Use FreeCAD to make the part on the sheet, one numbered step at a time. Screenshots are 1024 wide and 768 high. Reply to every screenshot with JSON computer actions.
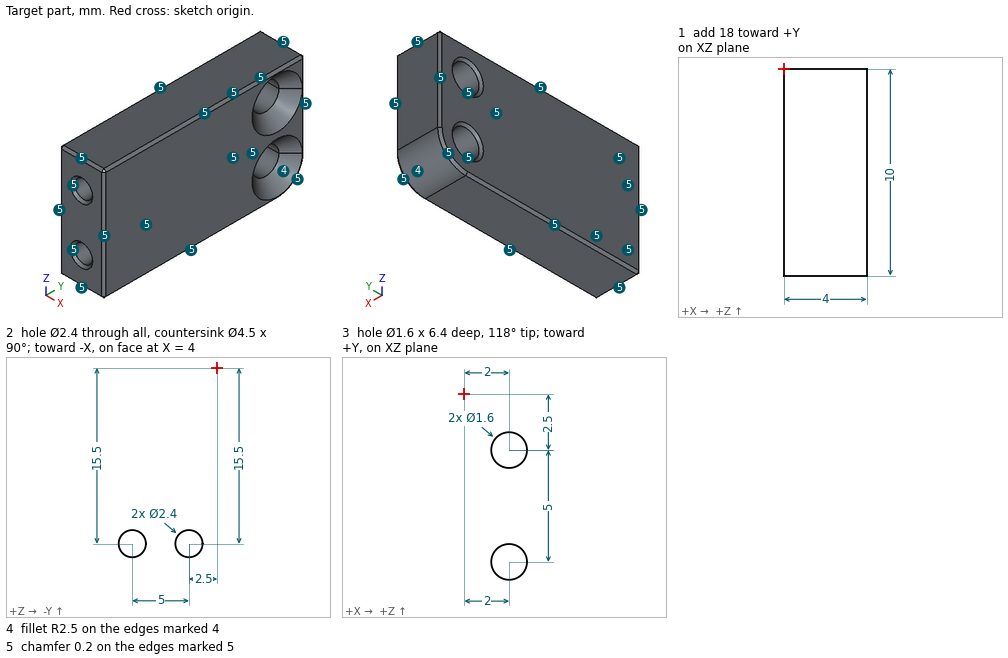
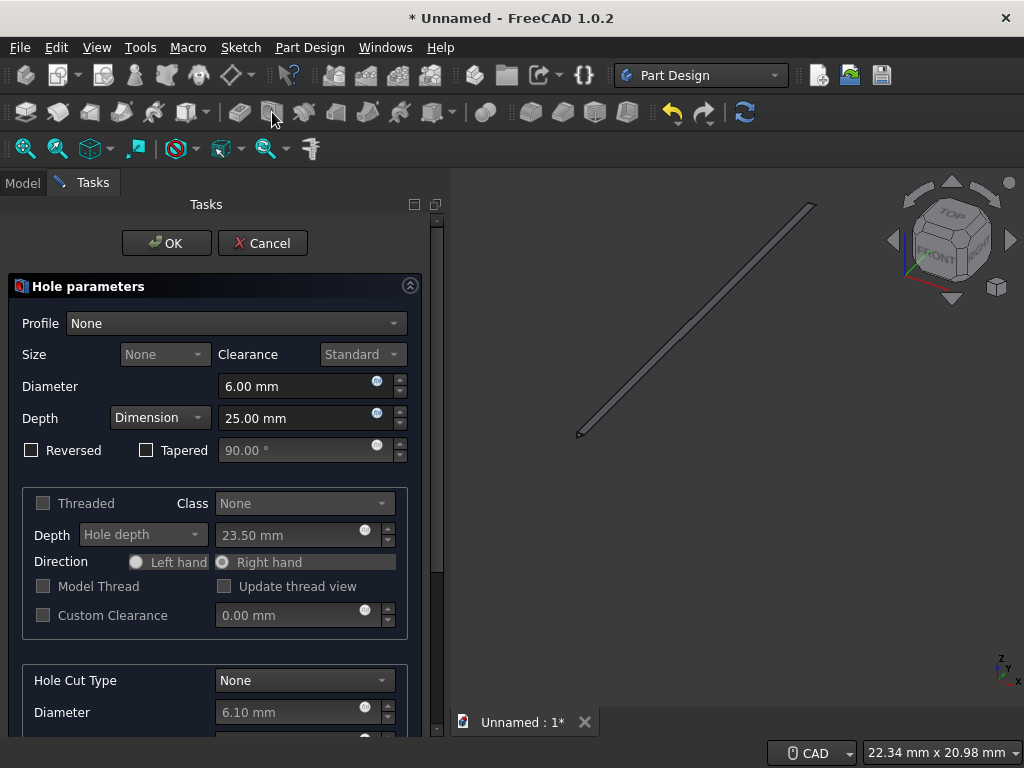
{"action": "triple_click", "coordinate": [305, 386]}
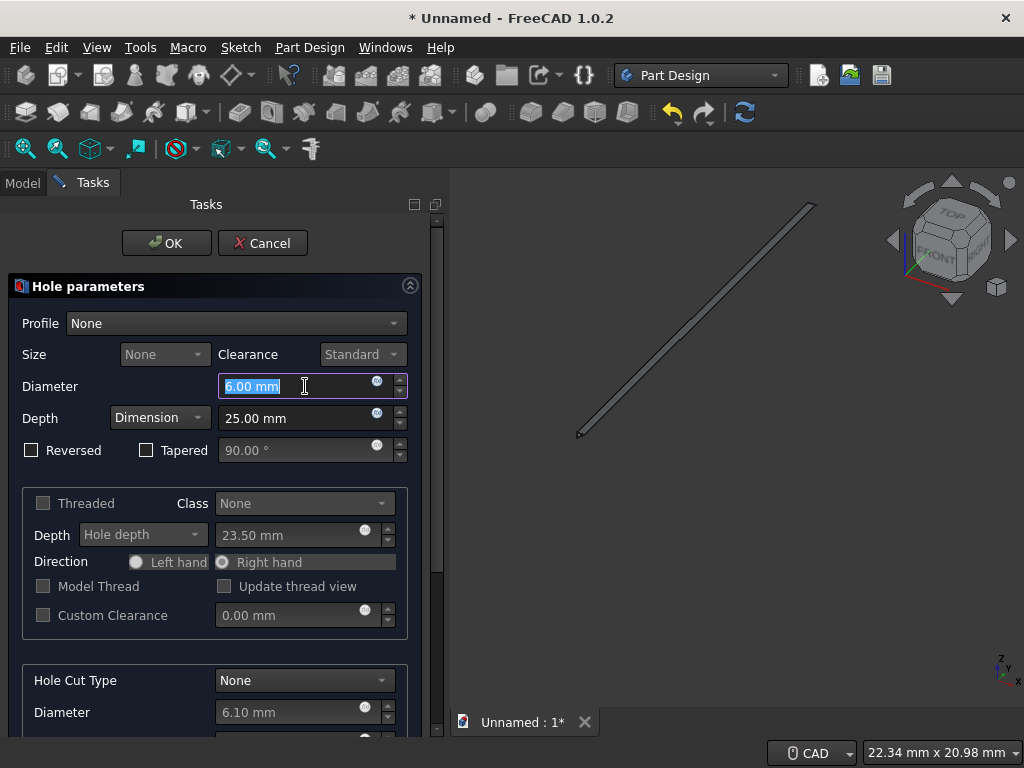
{"action": "type", "text": "1.6"}
{"action": "key", "text": "Tab"}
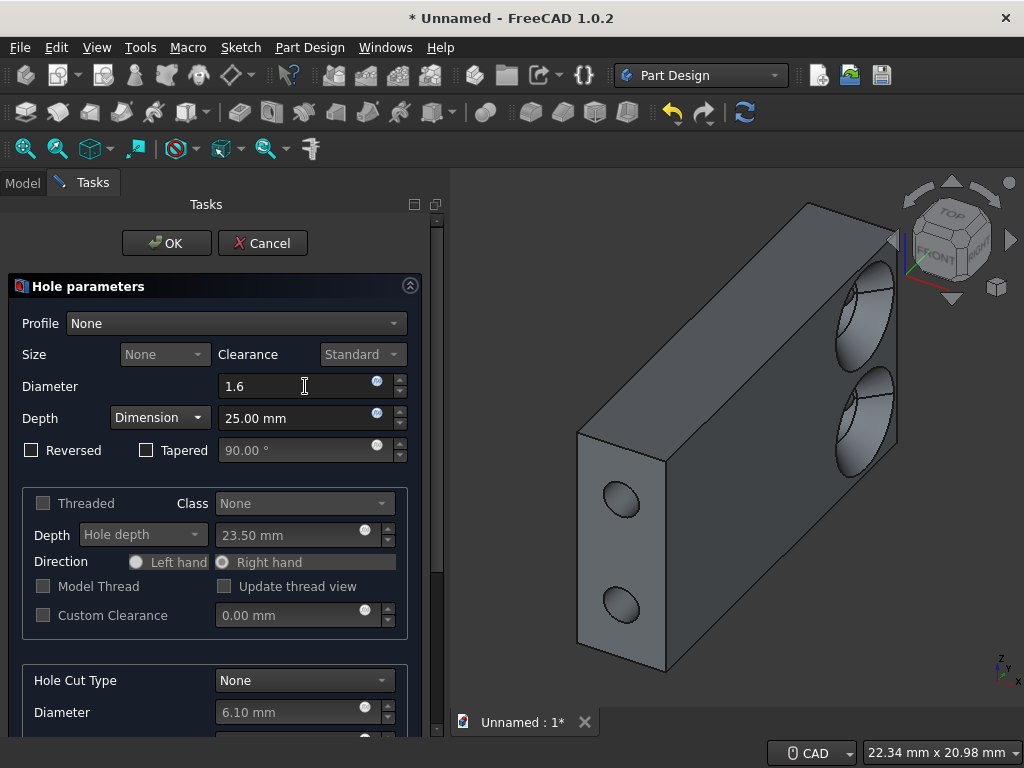
{"action": "triple_click", "coordinate": [305, 418]}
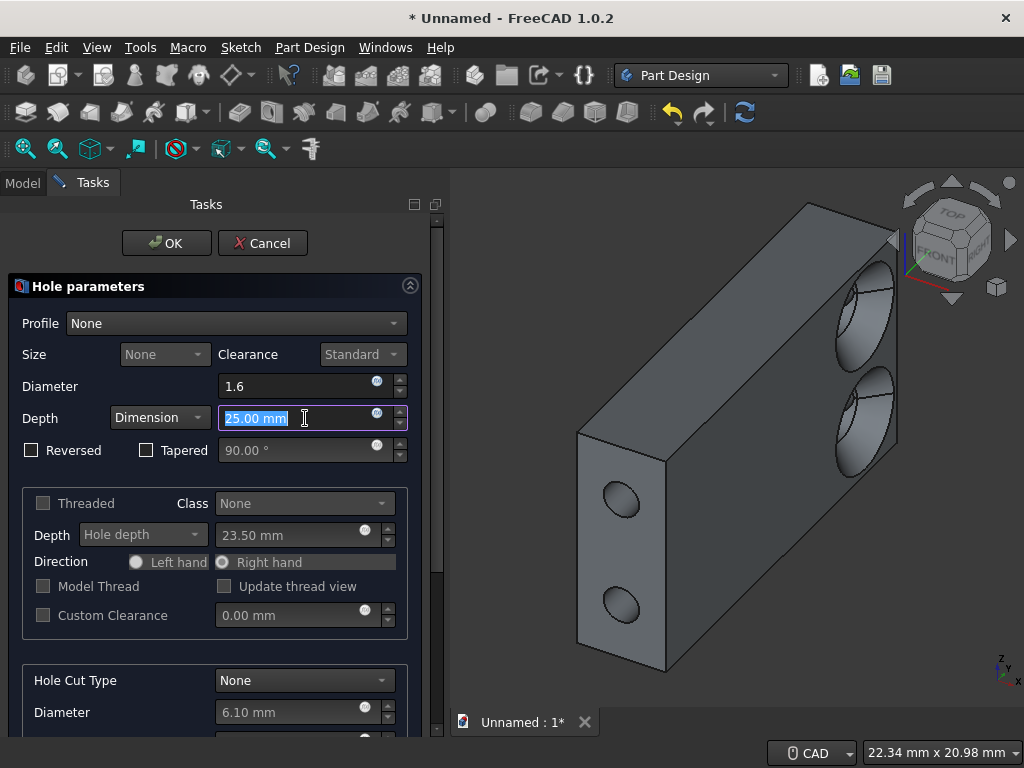
{"action": "type", "text": "6.4"}
{"action": "key", "text": "Tab"}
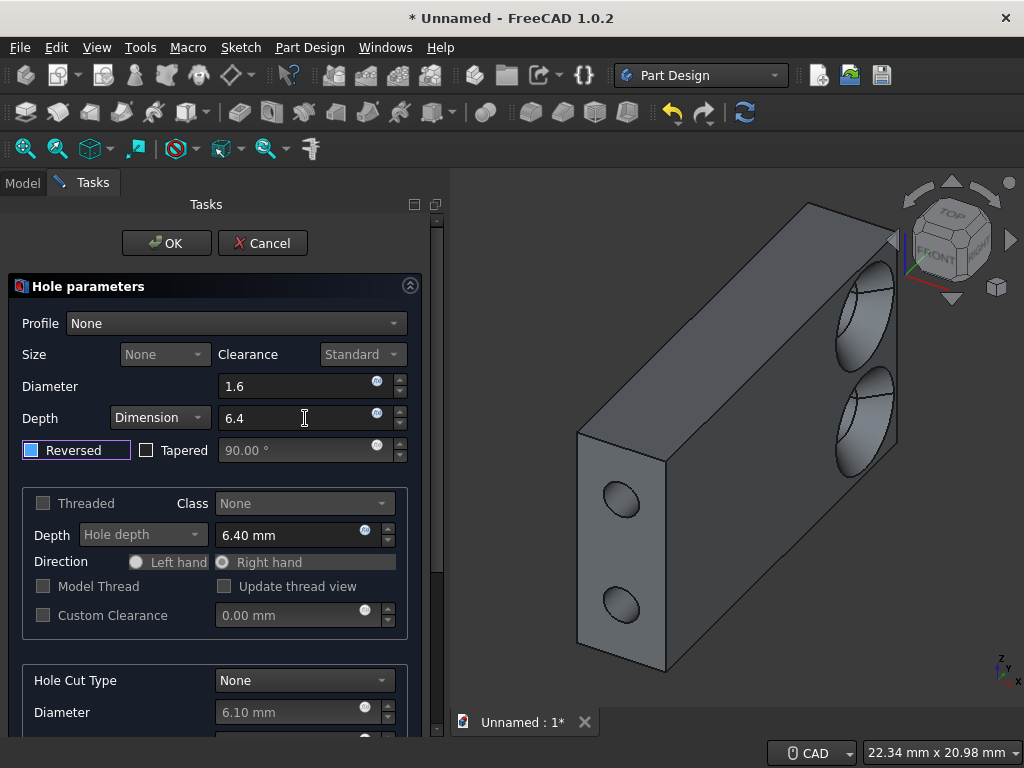
{"action": "left_click", "coordinate": [167, 243]}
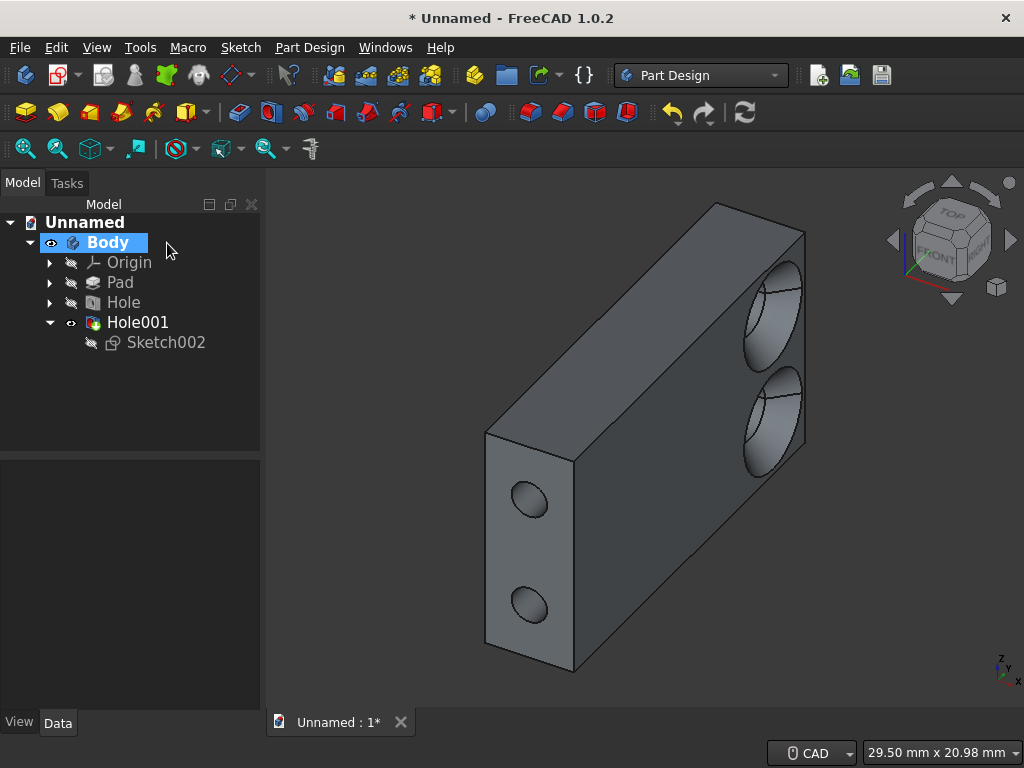
{"action": "key", "text": "0"}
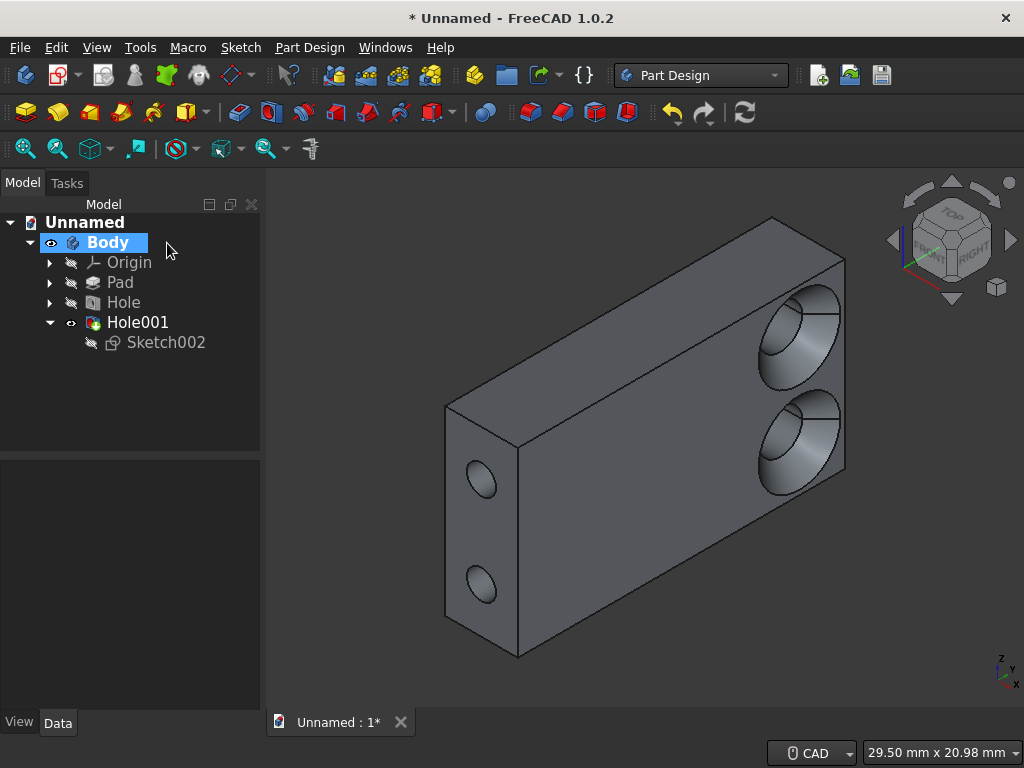
{"action": "key", "text": "2"}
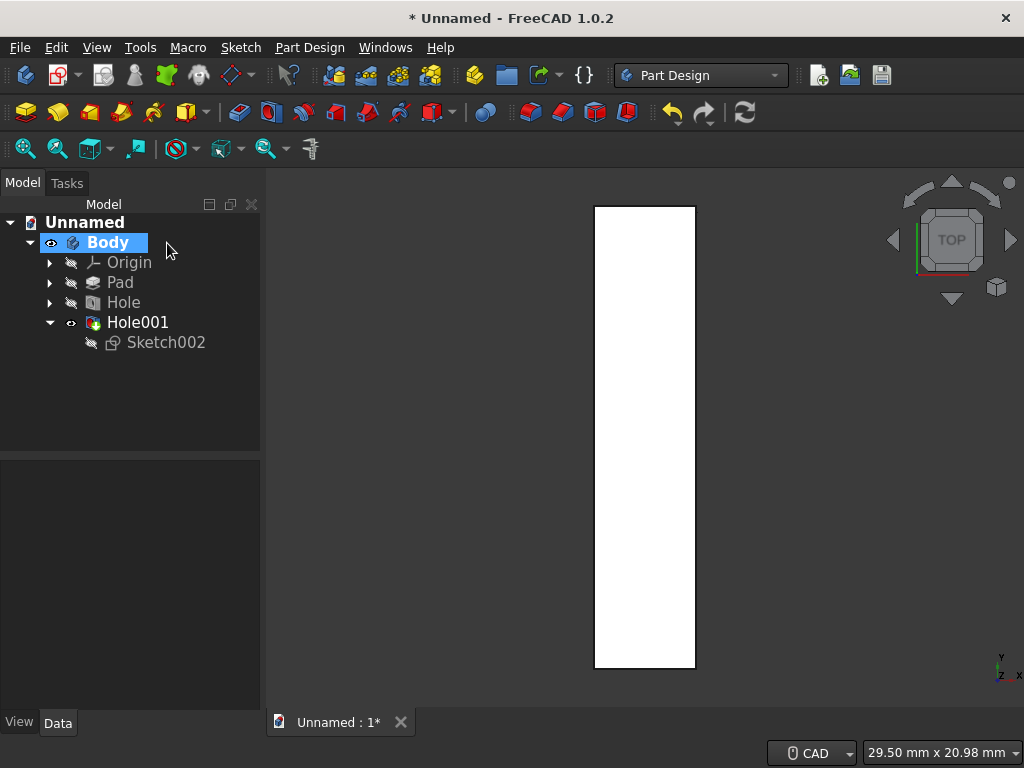
{"action": "key", "text": "1"}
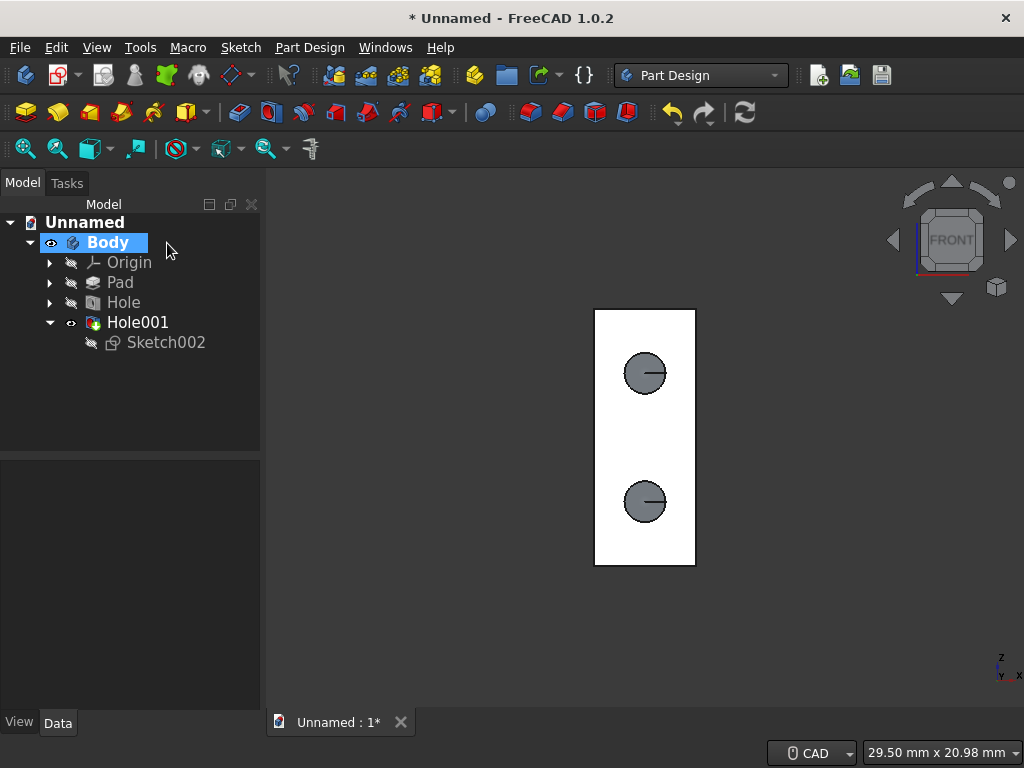
{"action": "key", "text": "3"}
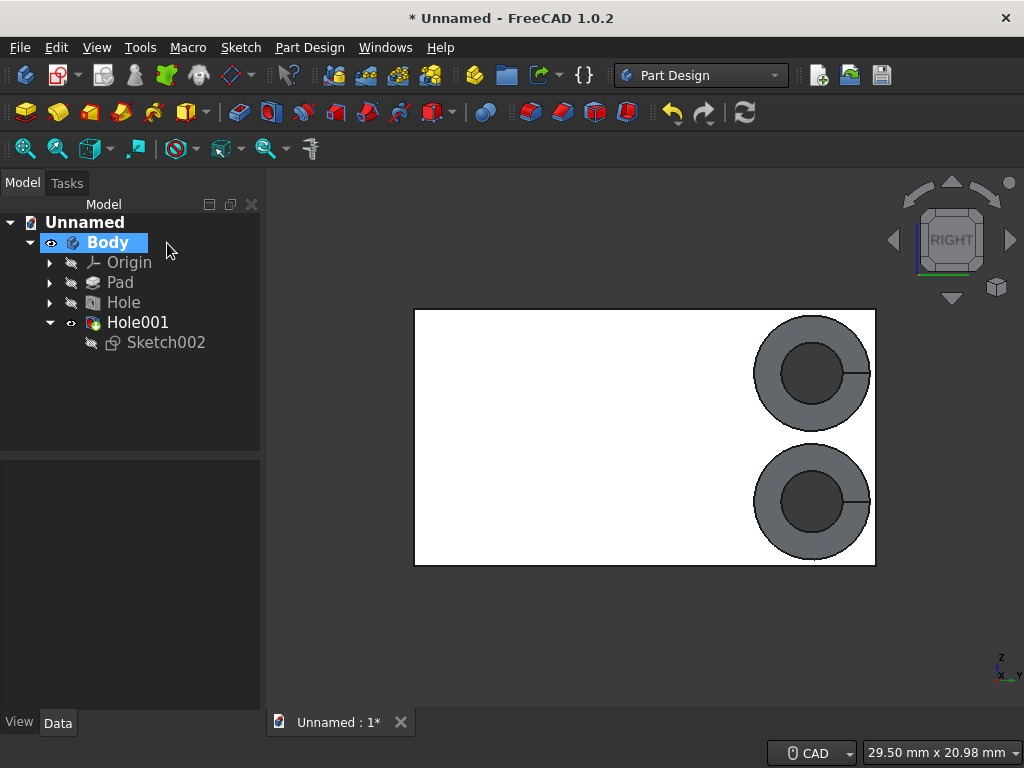
{"action": "key", "text": "5"}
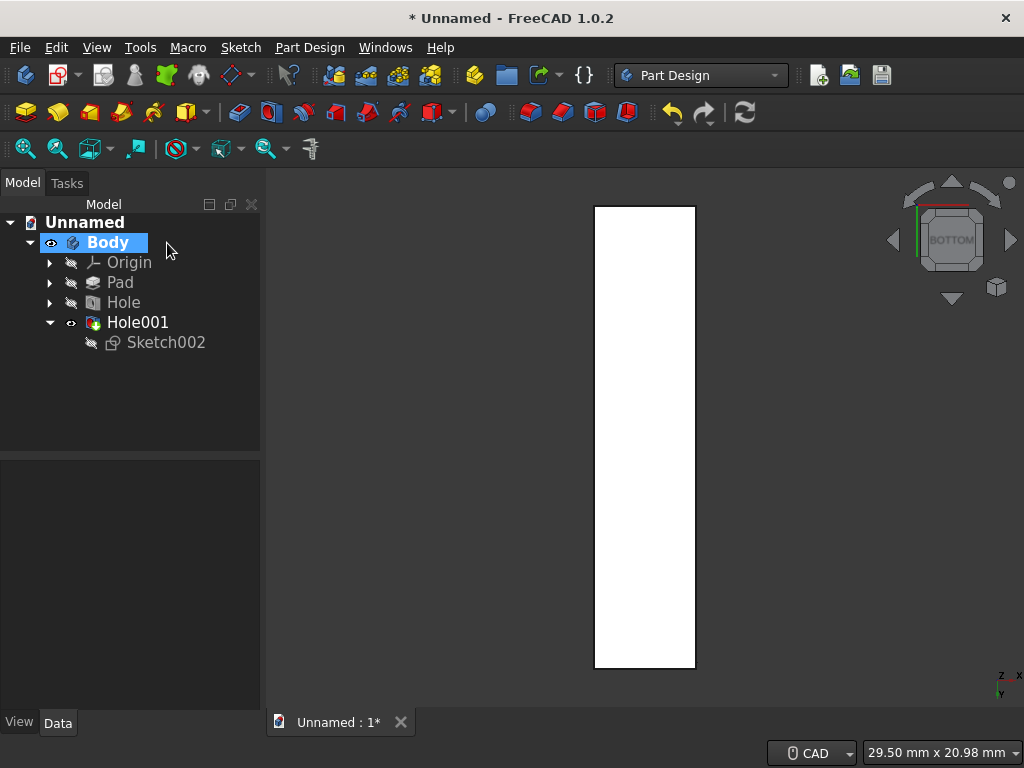
{"action": "key", "text": "4"}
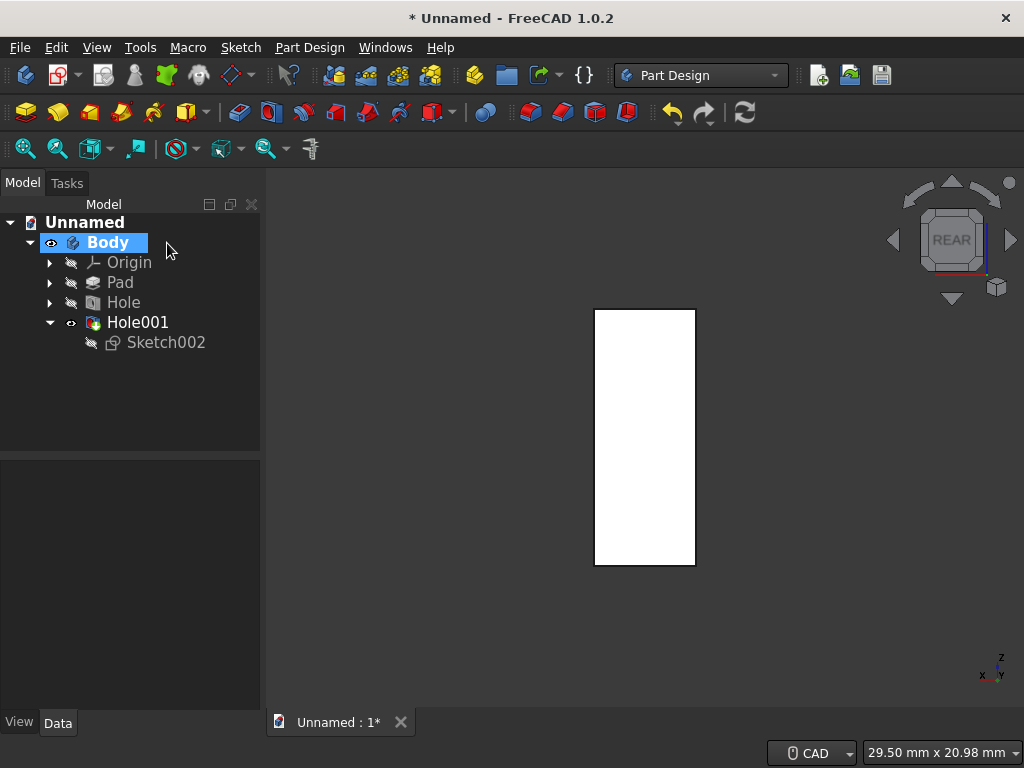
{"action": "left_click", "coordinate": [645, 565]}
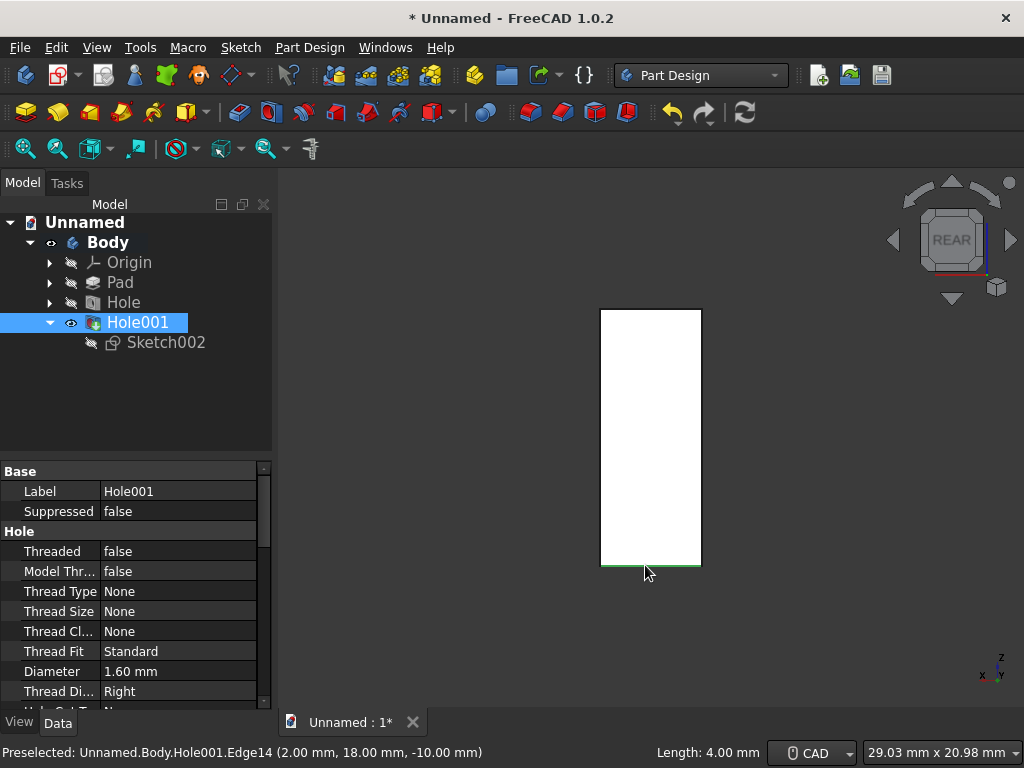
{"action": "left_click", "coordinate": [532, 112]}